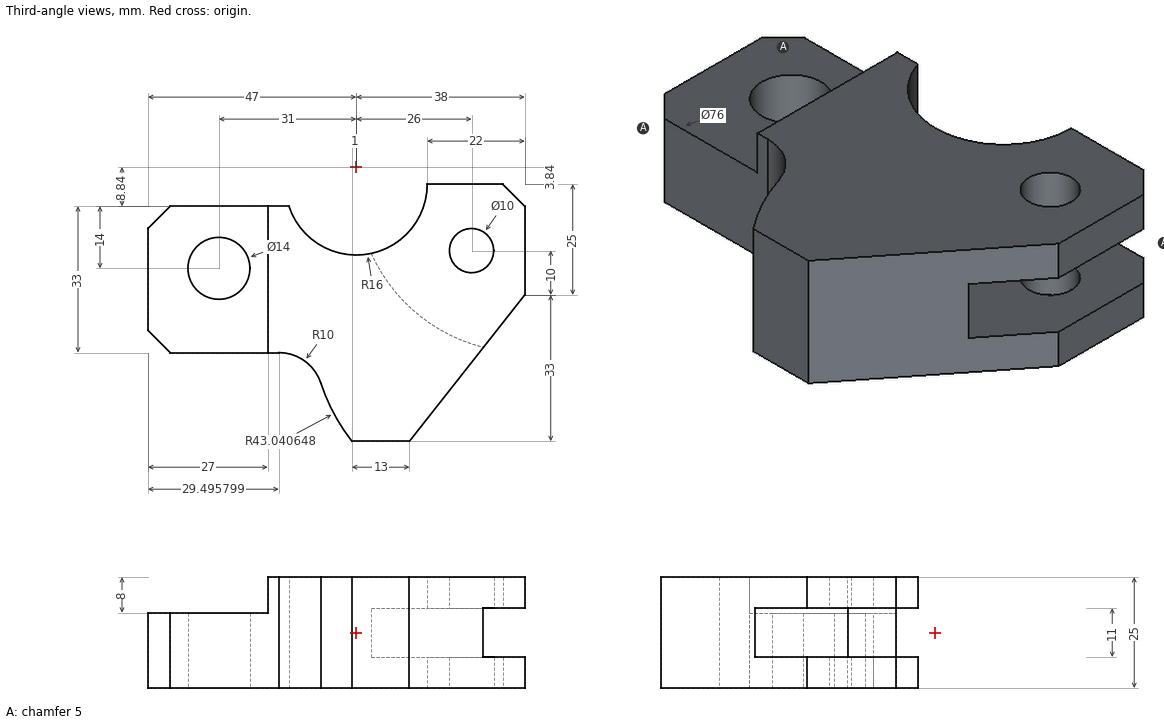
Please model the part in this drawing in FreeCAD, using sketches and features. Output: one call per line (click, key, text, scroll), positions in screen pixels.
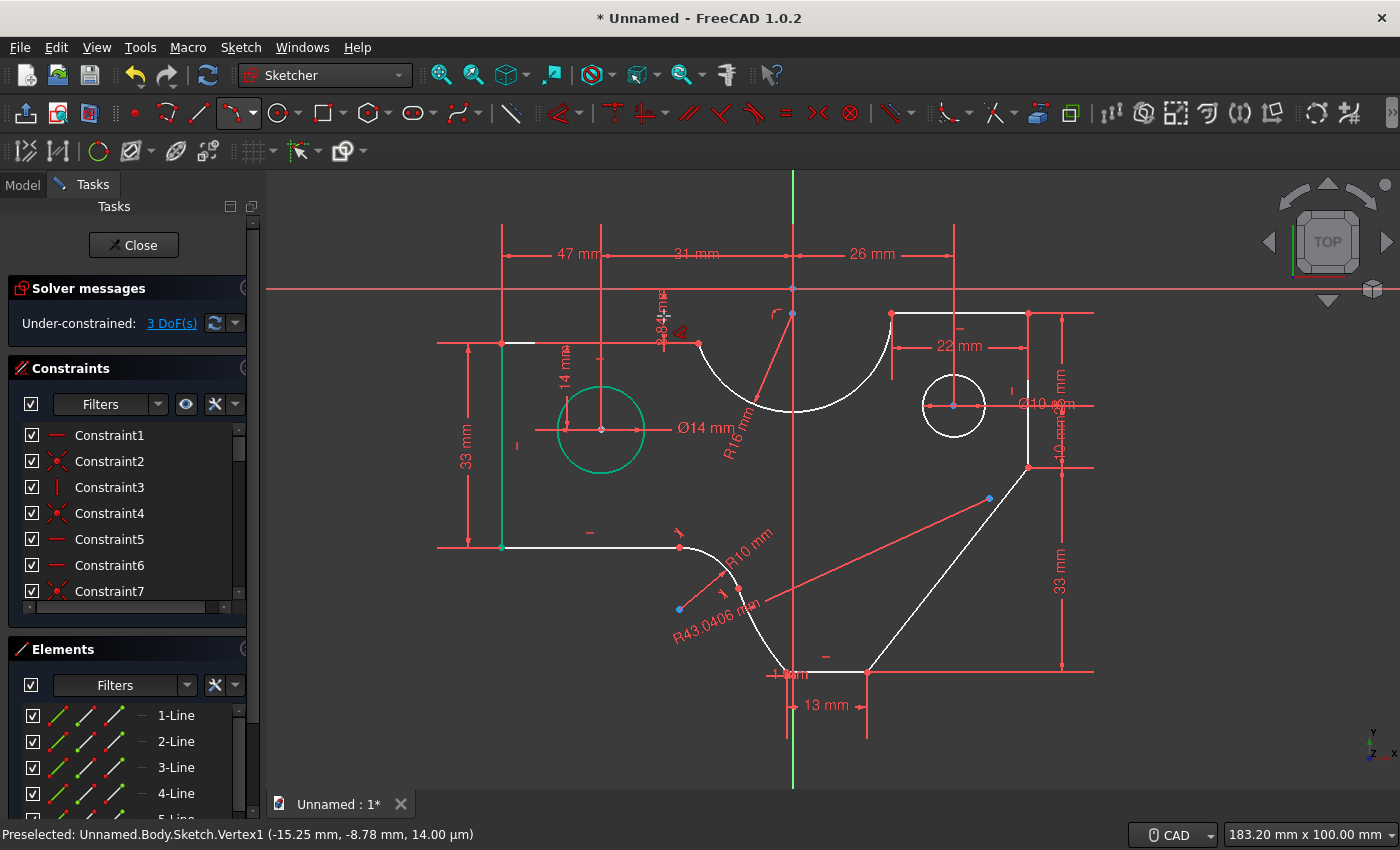
scroll(1028, 313, up, 3)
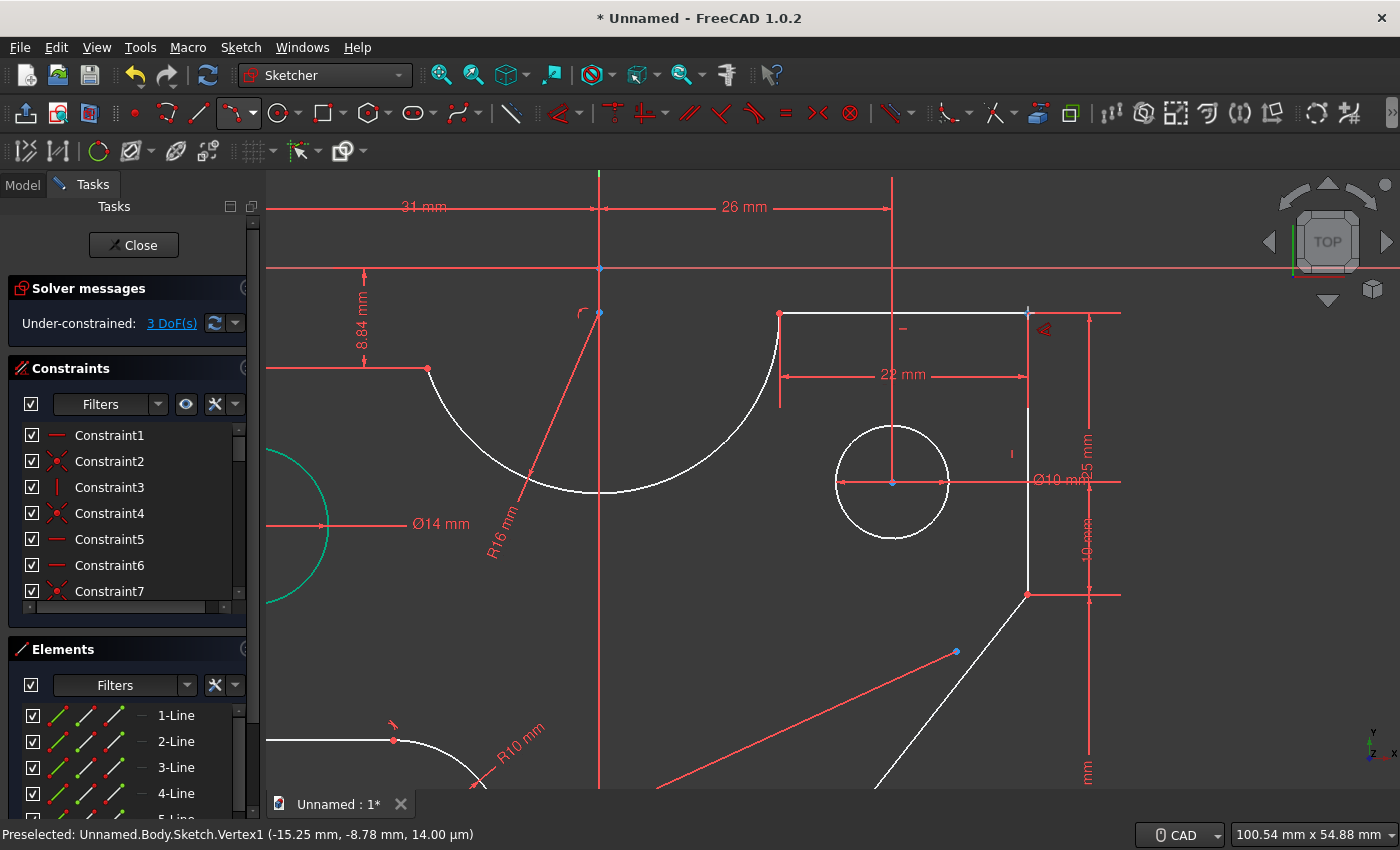
click(1028, 313)
click(1062, 291)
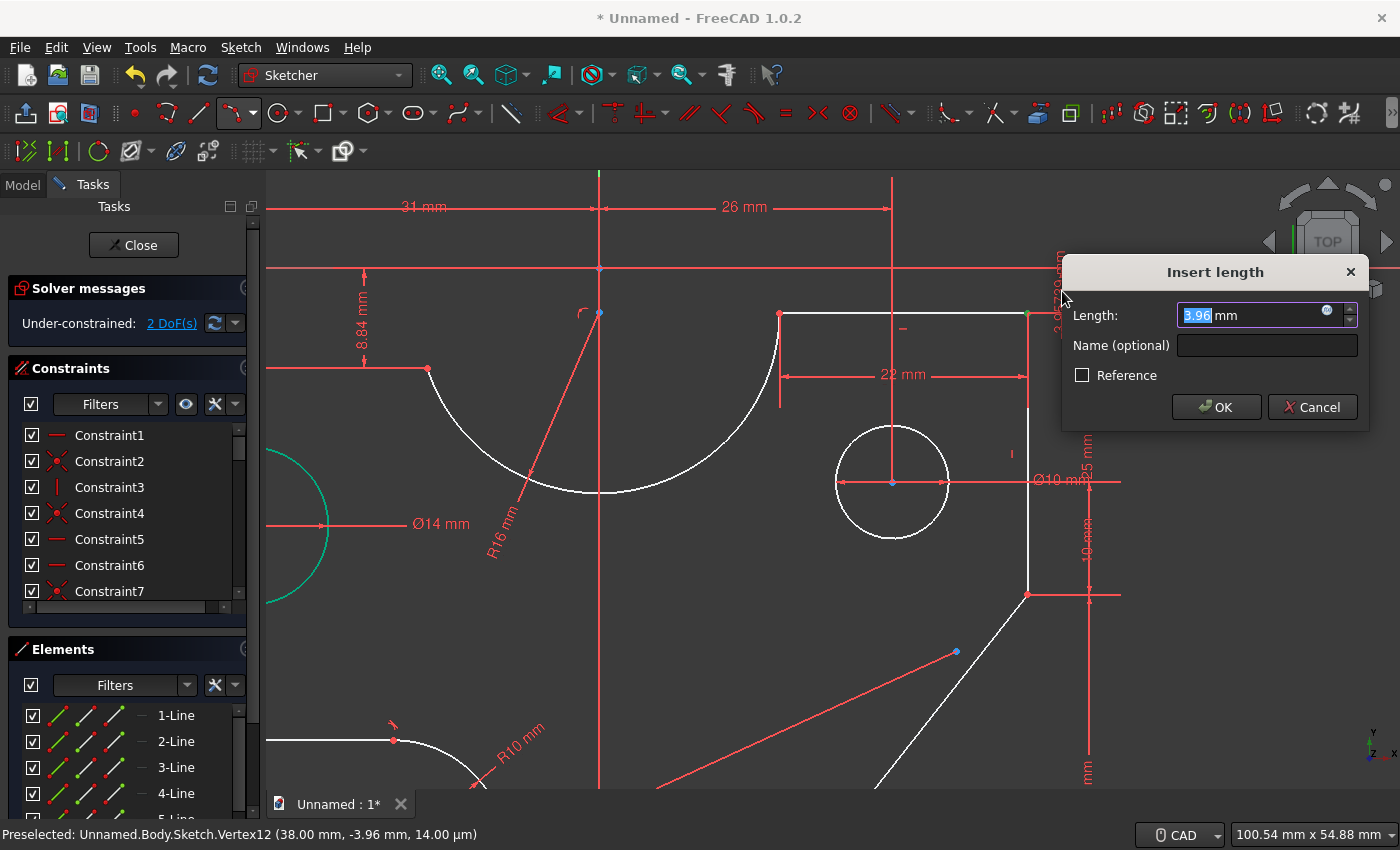
text(3.84)
key(Return)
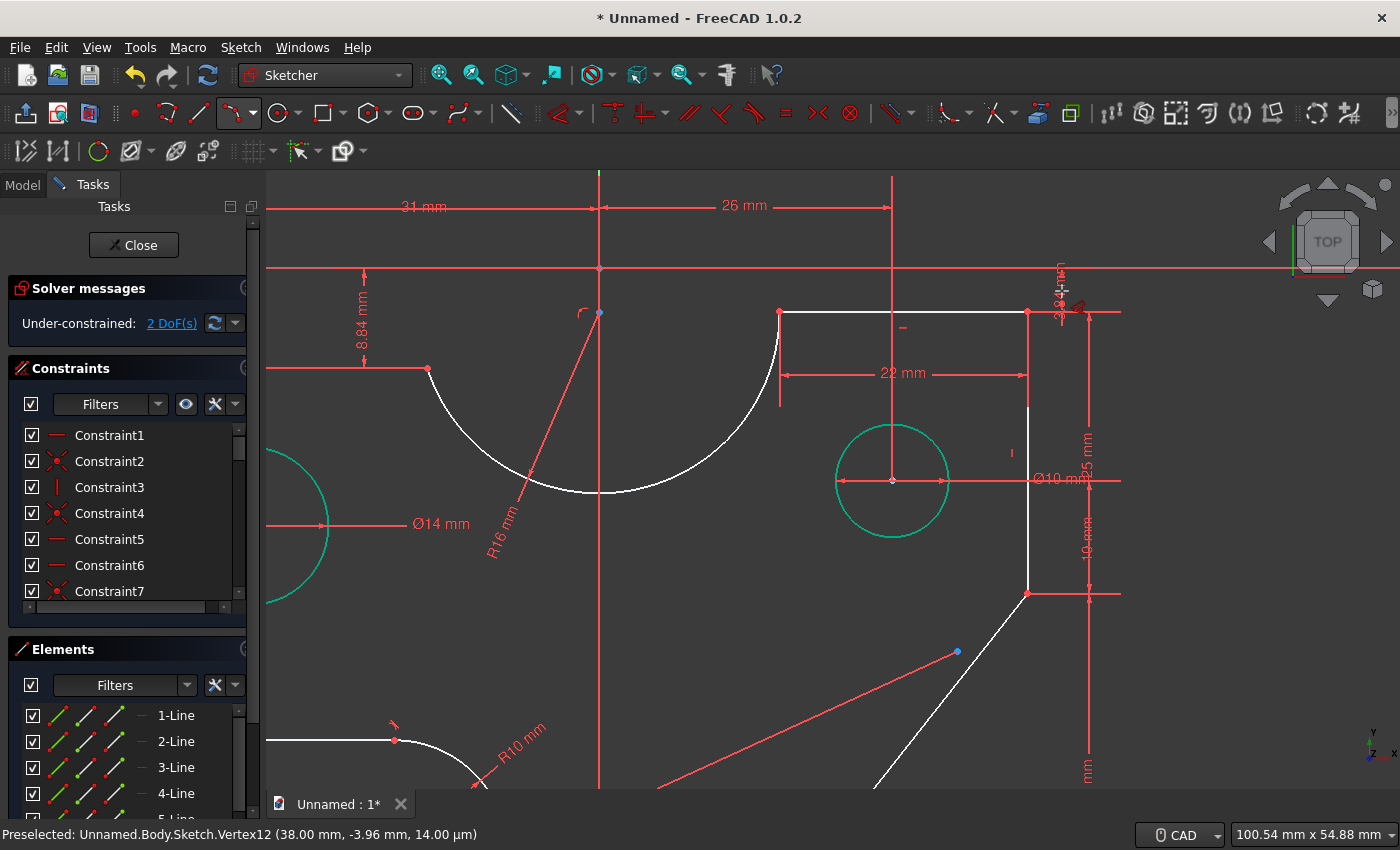
click(599, 313)
click(633, 291)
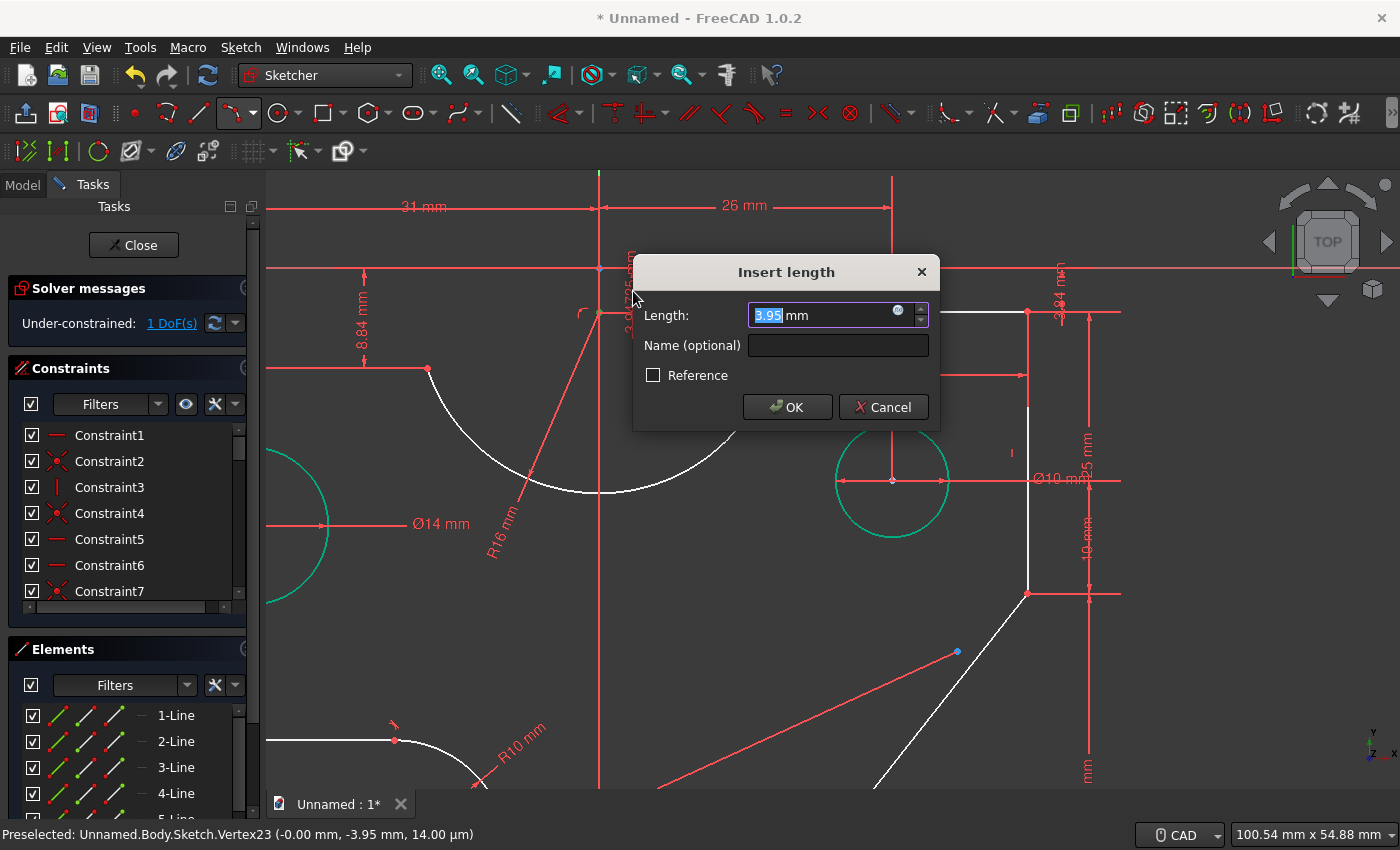
text(3.84)
key(Return)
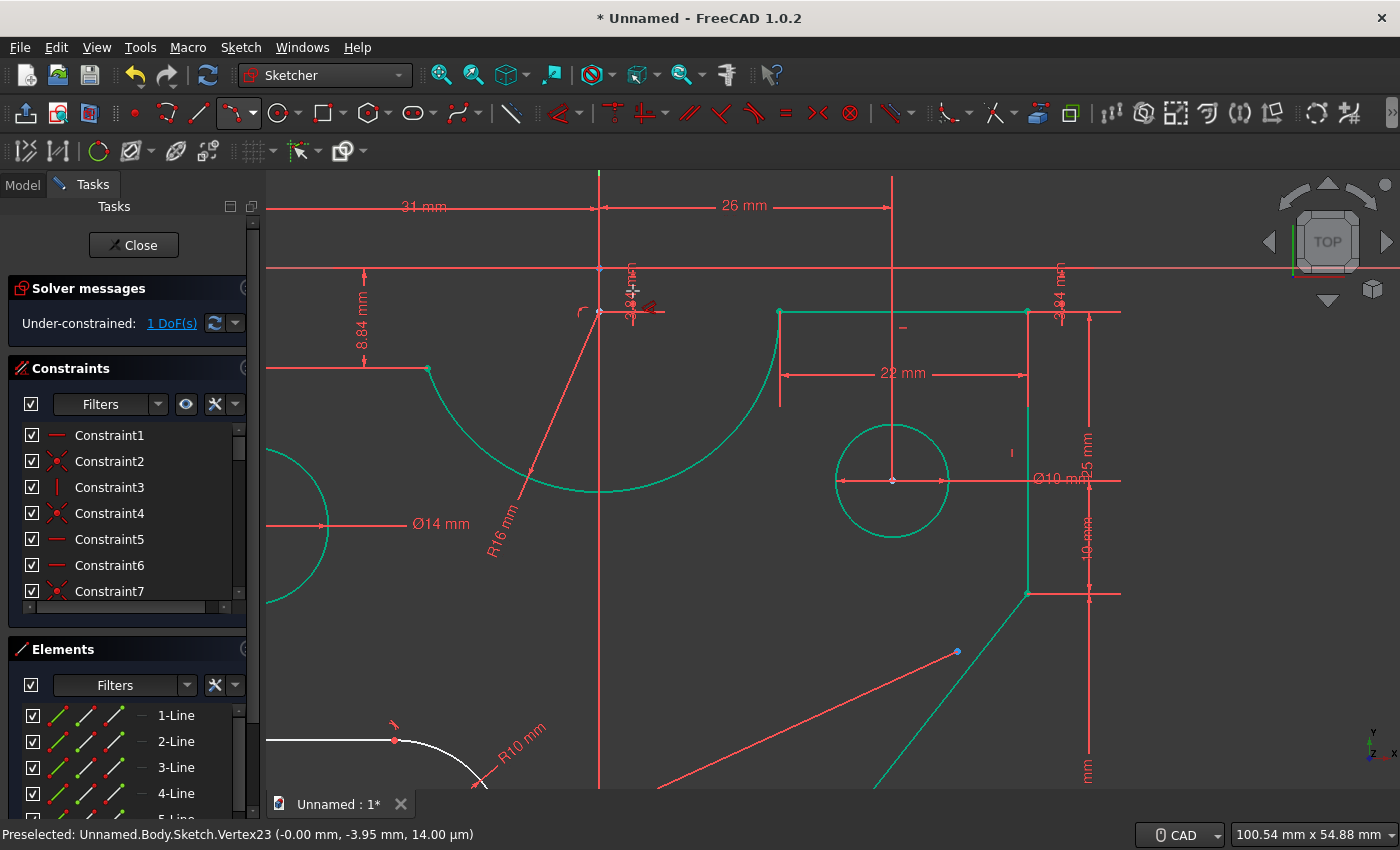
click(297, 740)
click(344, 706)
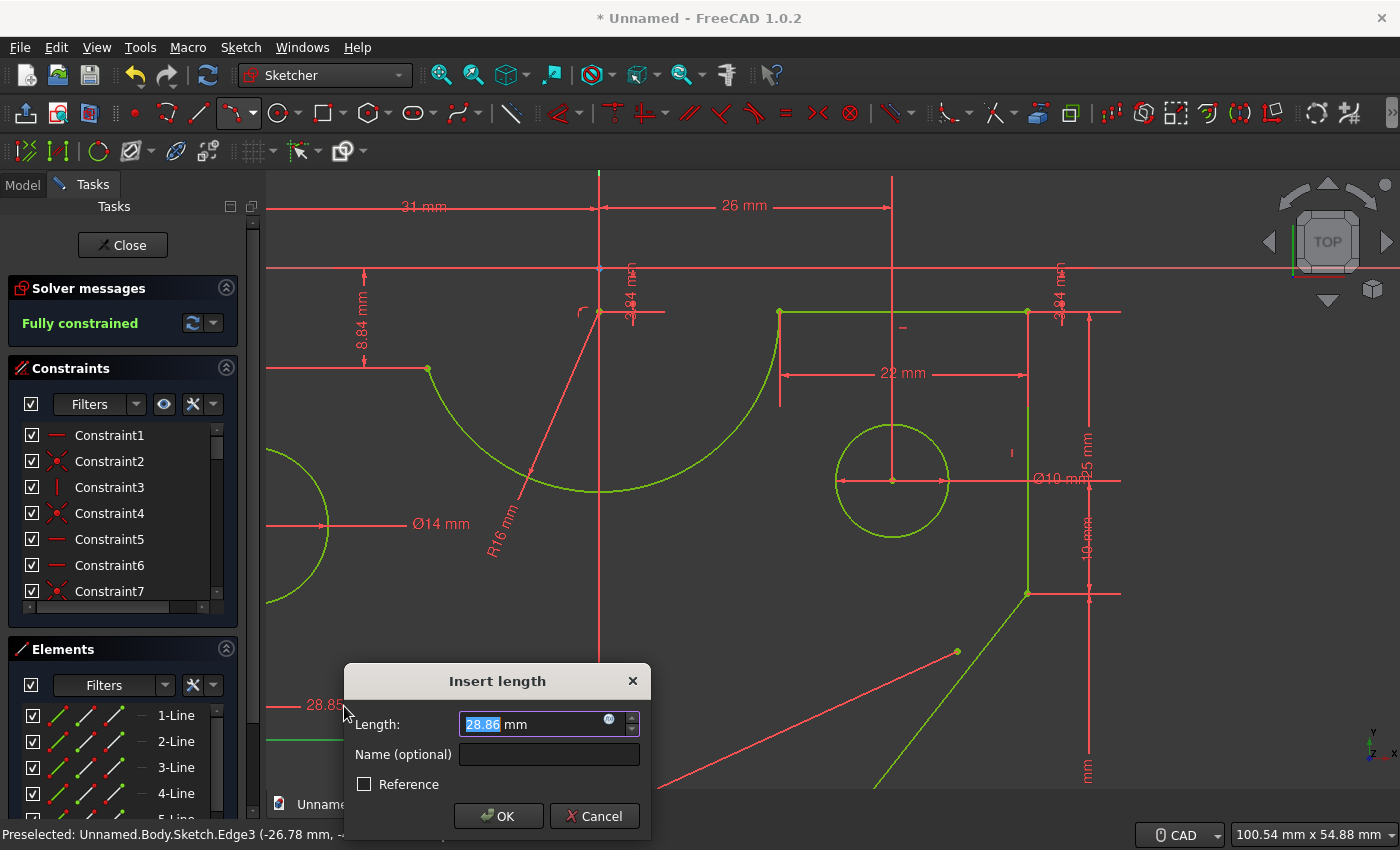
text(29.495799)
key(Return)
key(Escape)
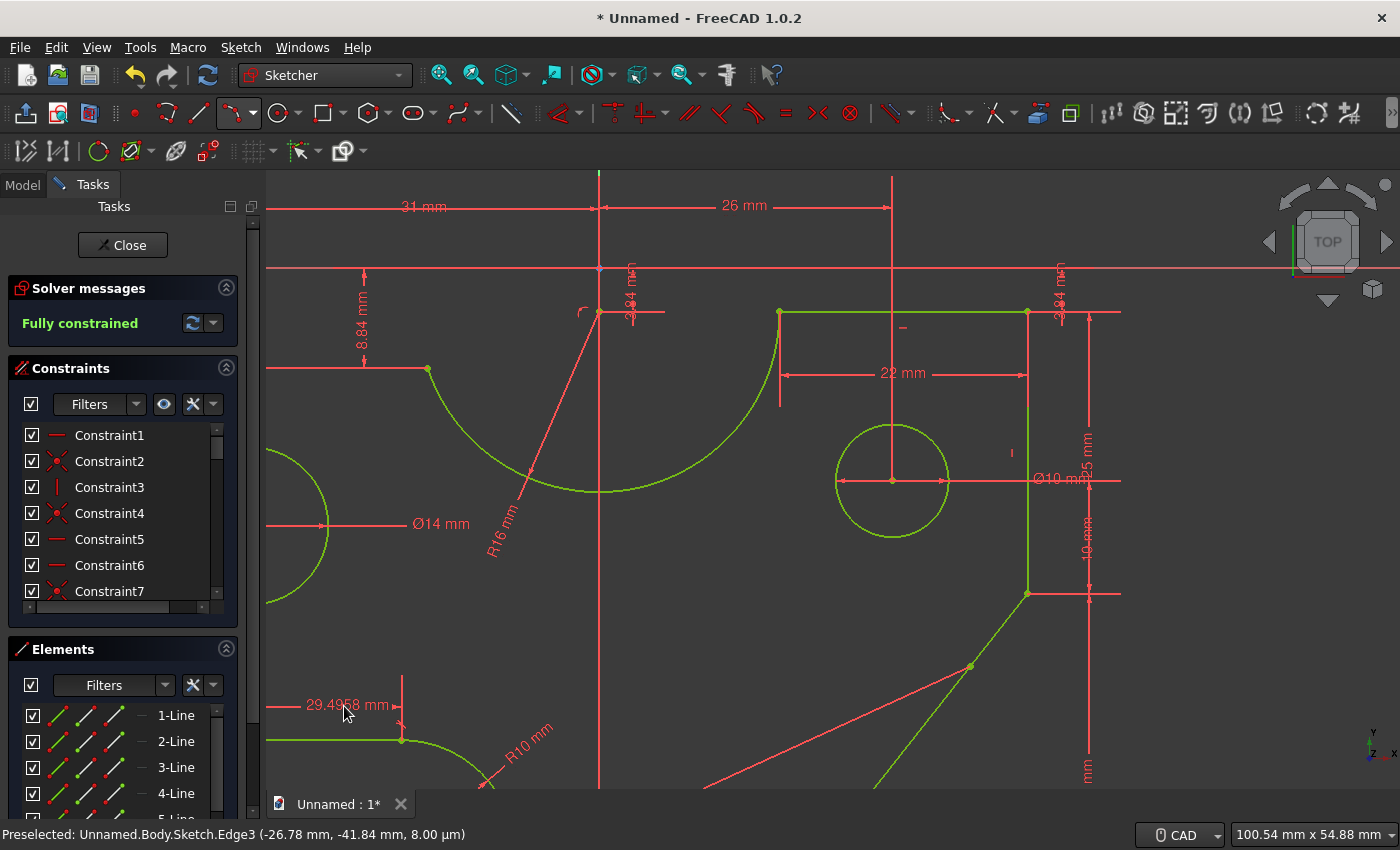
click(123, 245)